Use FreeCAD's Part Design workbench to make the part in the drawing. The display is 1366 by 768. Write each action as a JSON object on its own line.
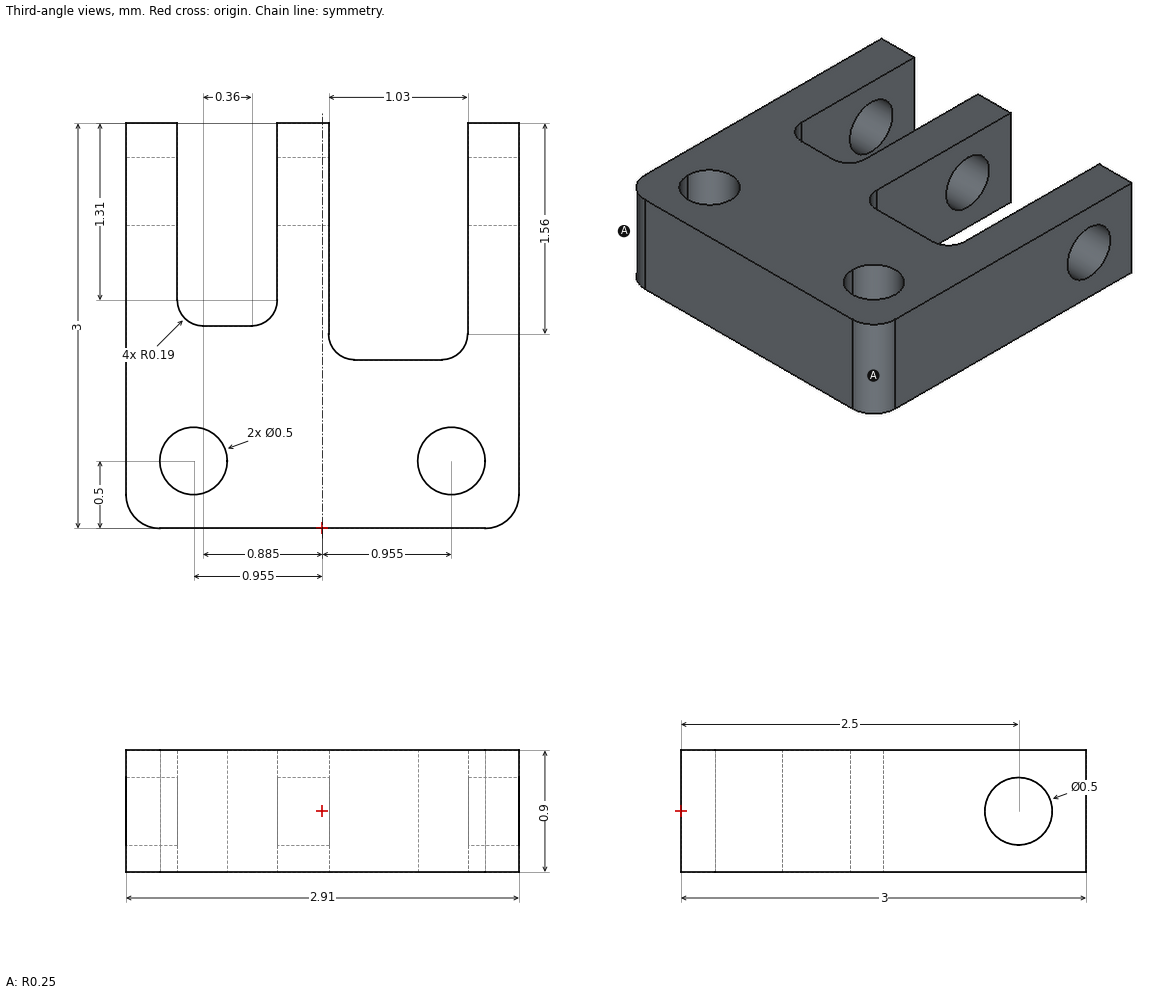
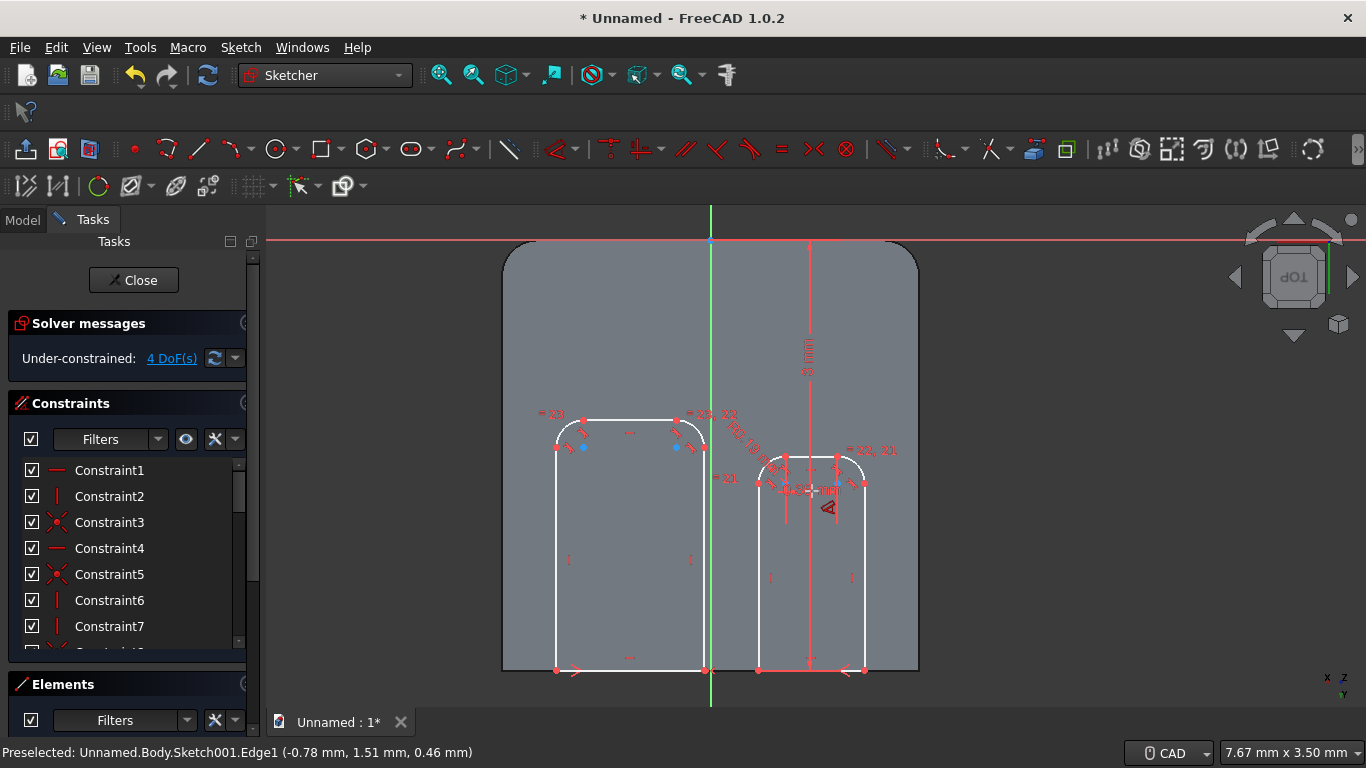
{"action": "left_click", "coordinate": [759, 540]}
{"action": "left_click", "coordinate": [793, 577]}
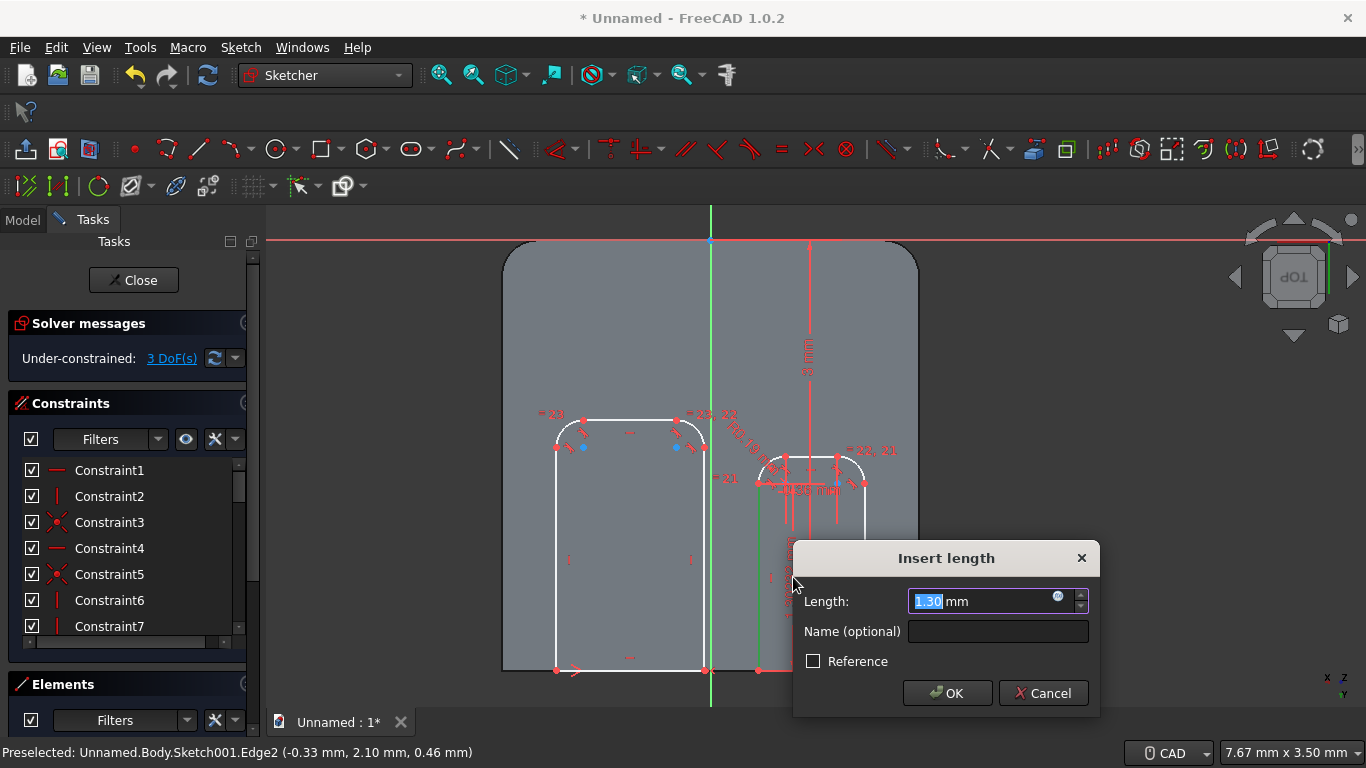
{"action": "type", "text": "1.31"}
{"action": "key", "text": "Return"}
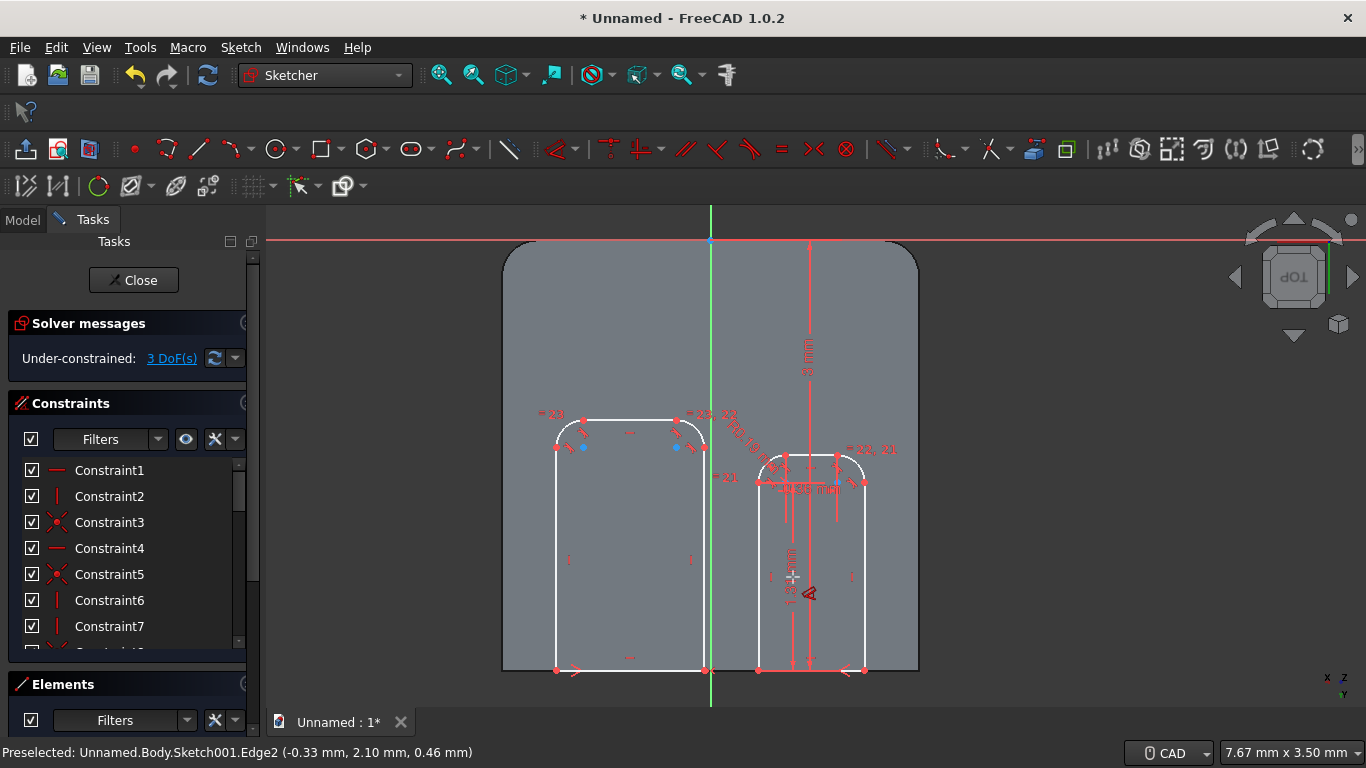
{"action": "left_click", "coordinate": [556, 514]}
{"action": "left_click", "coordinate": [522, 559]}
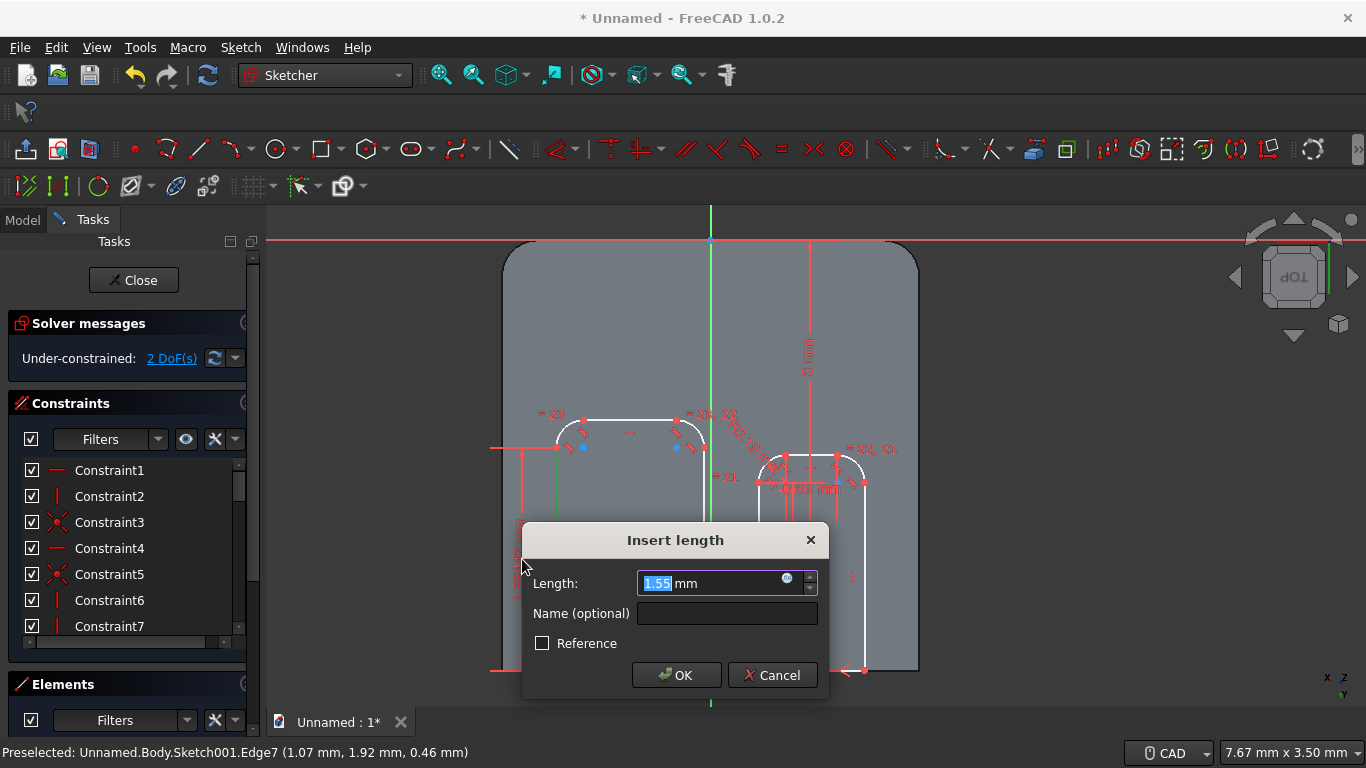
{"action": "type", "text": "1.56"}
{"action": "key", "text": "Return"}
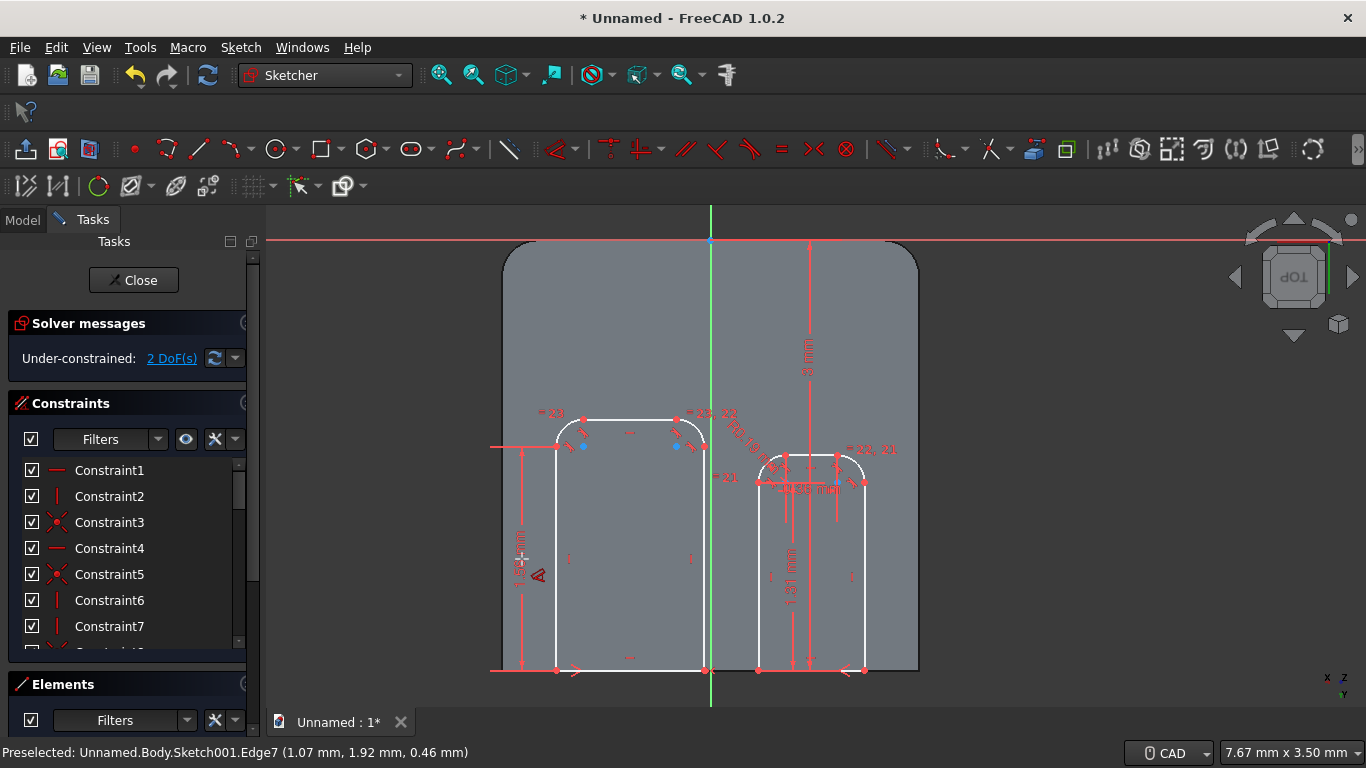
{"action": "left_click", "coordinate": [601, 671]}
{"action": "left_click", "coordinate": [630, 637]}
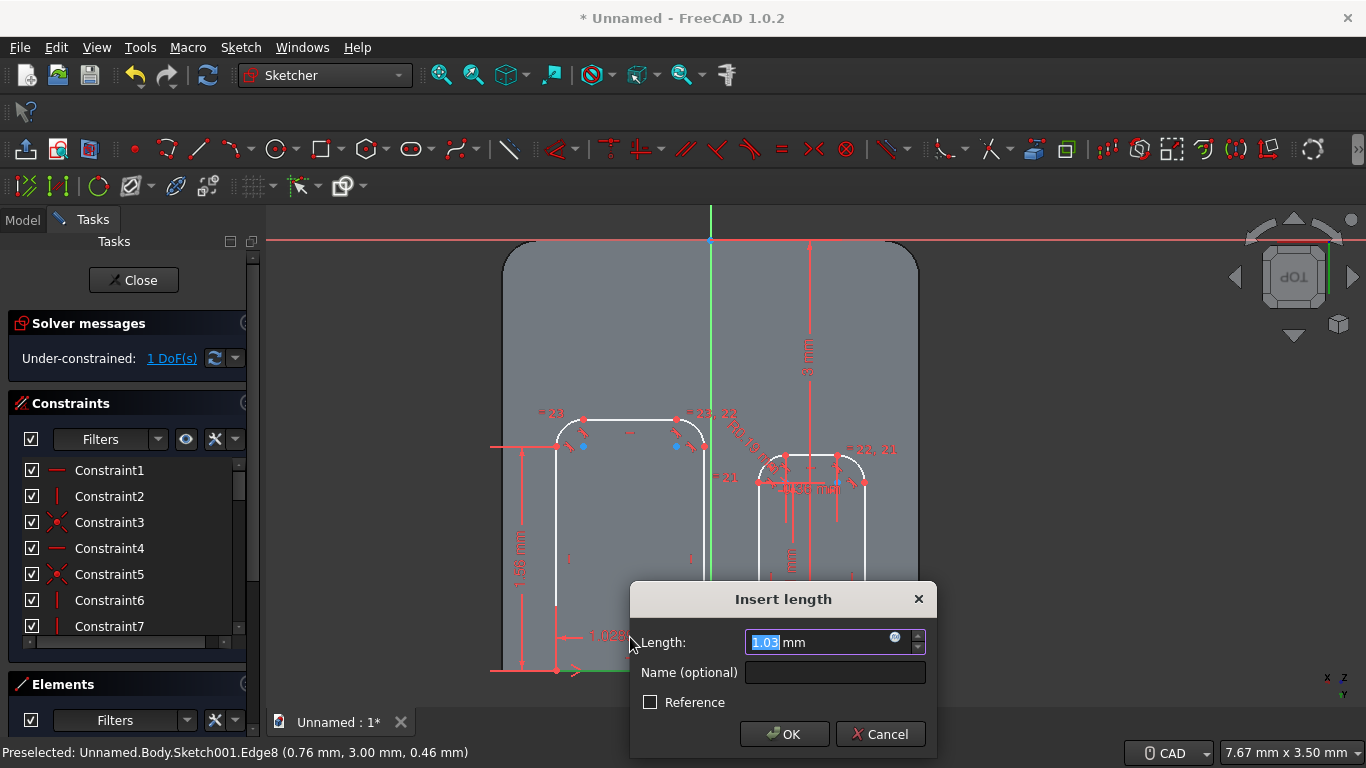
{"action": "type", "text": "1.03"}
{"action": "key", "text": "Return"}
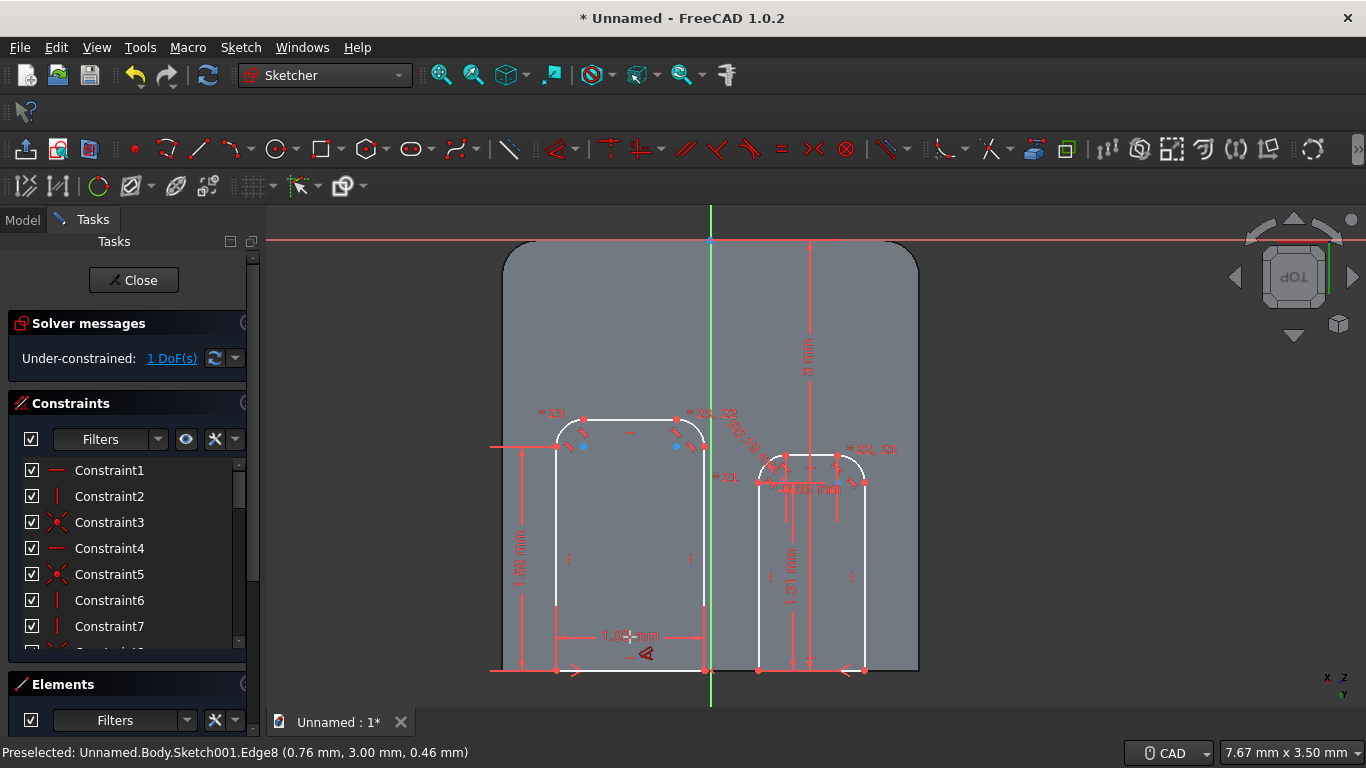
{"action": "left_click", "coordinate": [837, 455]}
{"action": "left_click", "coordinate": [730, 489]}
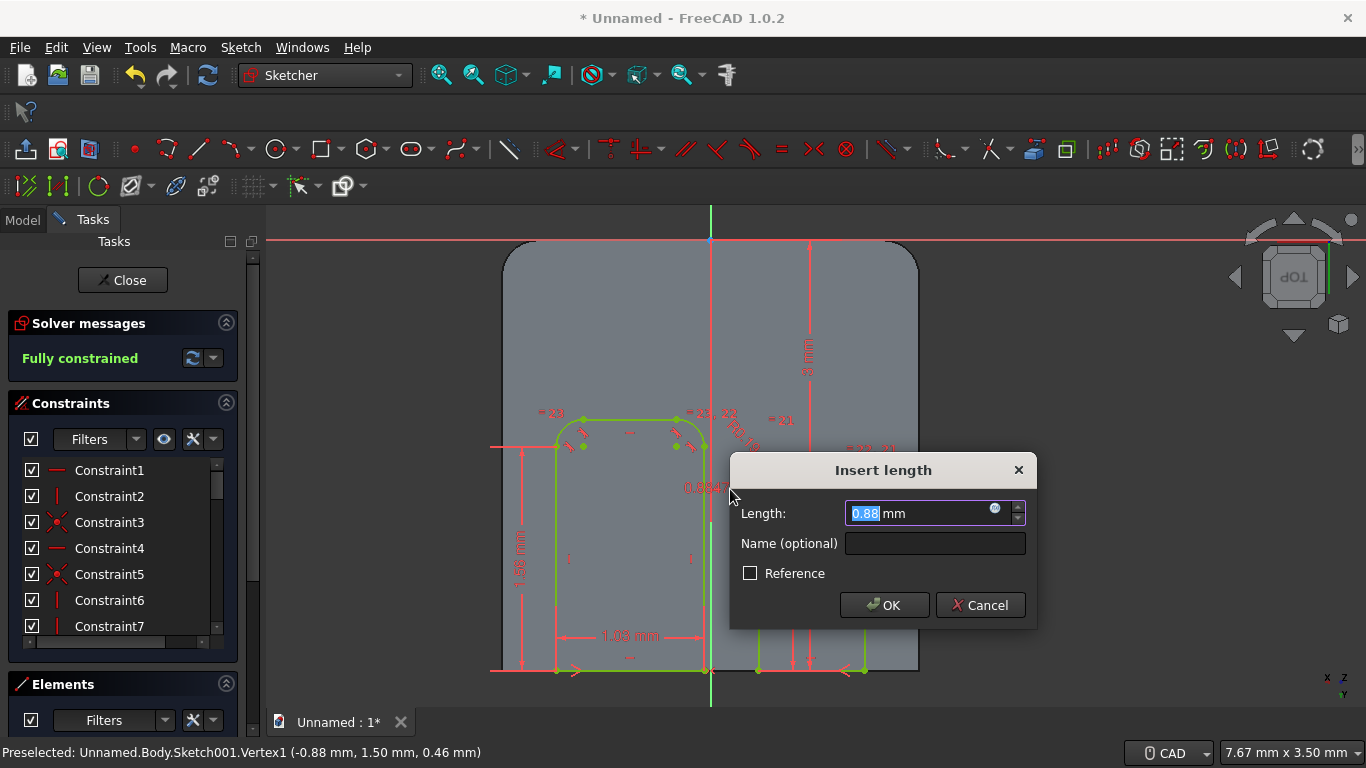
{"action": "type", "text": "0.885"}
{"action": "key", "text": "Return"}
{"action": "key", "text": "Escape"}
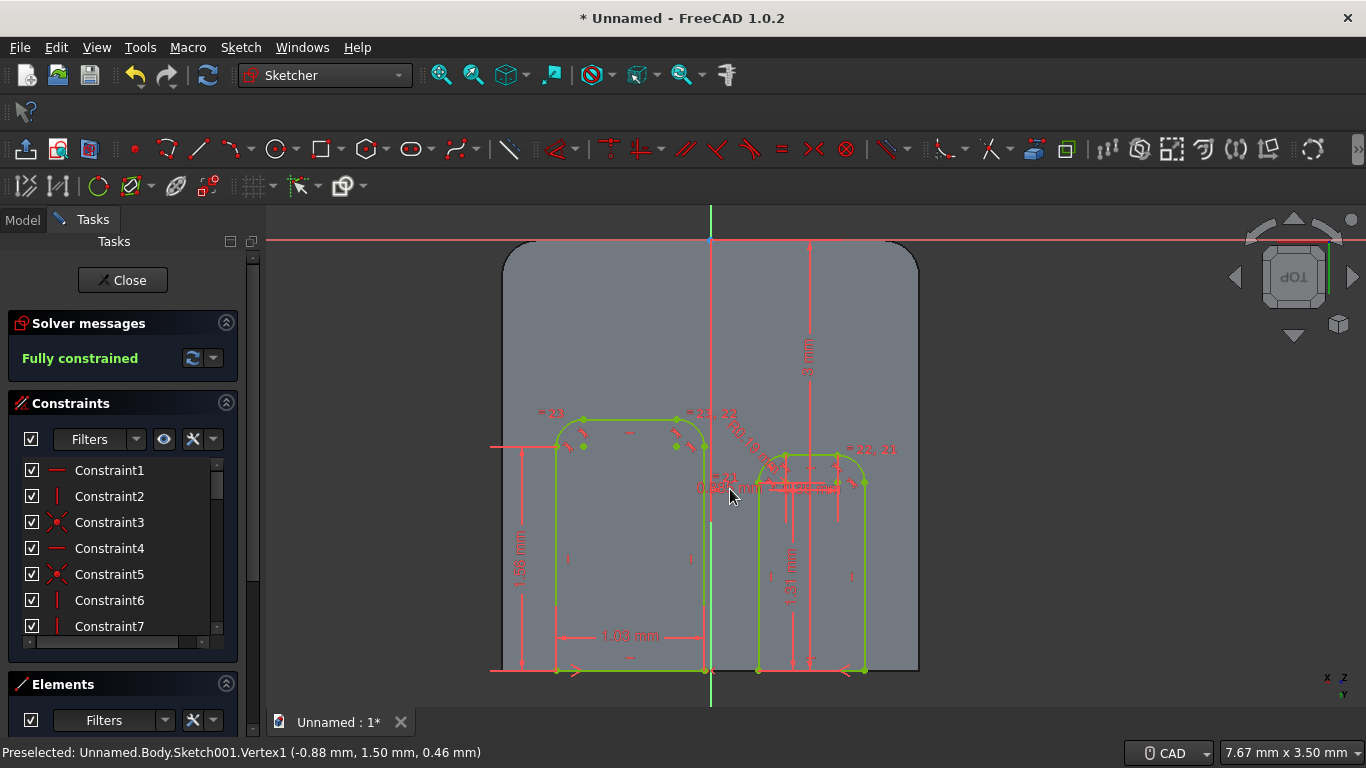
{"action": "left_click", "coordinate": [123, 280]}